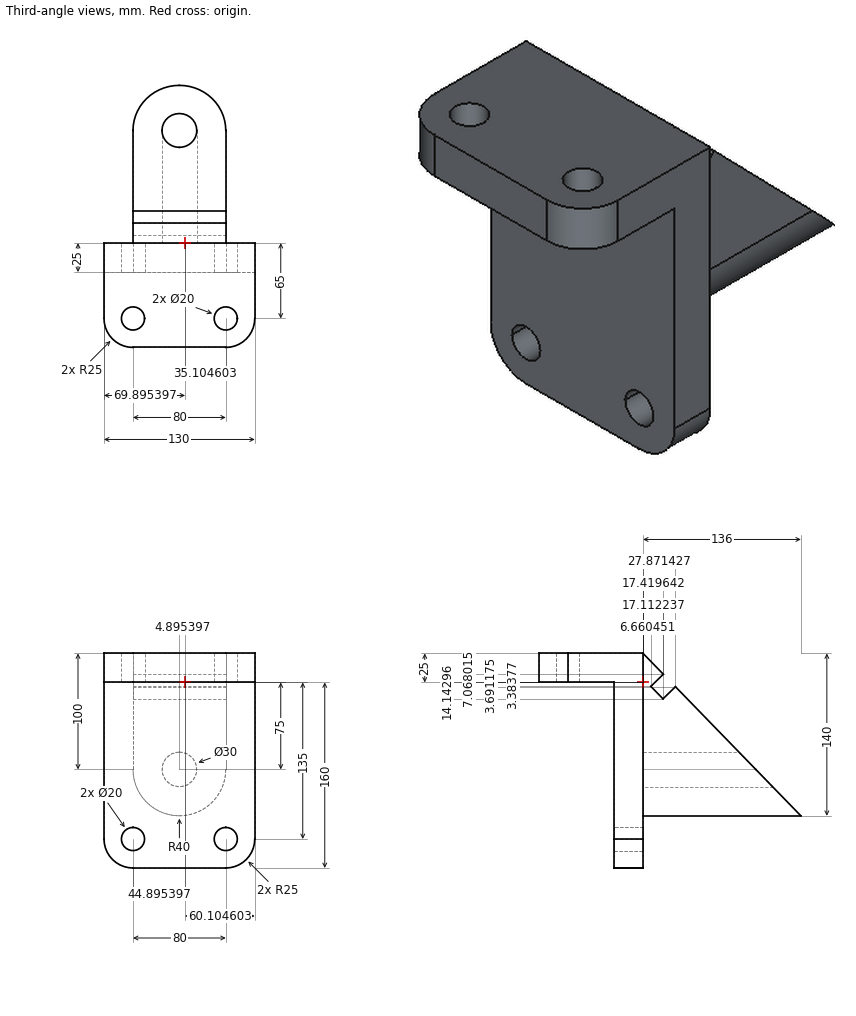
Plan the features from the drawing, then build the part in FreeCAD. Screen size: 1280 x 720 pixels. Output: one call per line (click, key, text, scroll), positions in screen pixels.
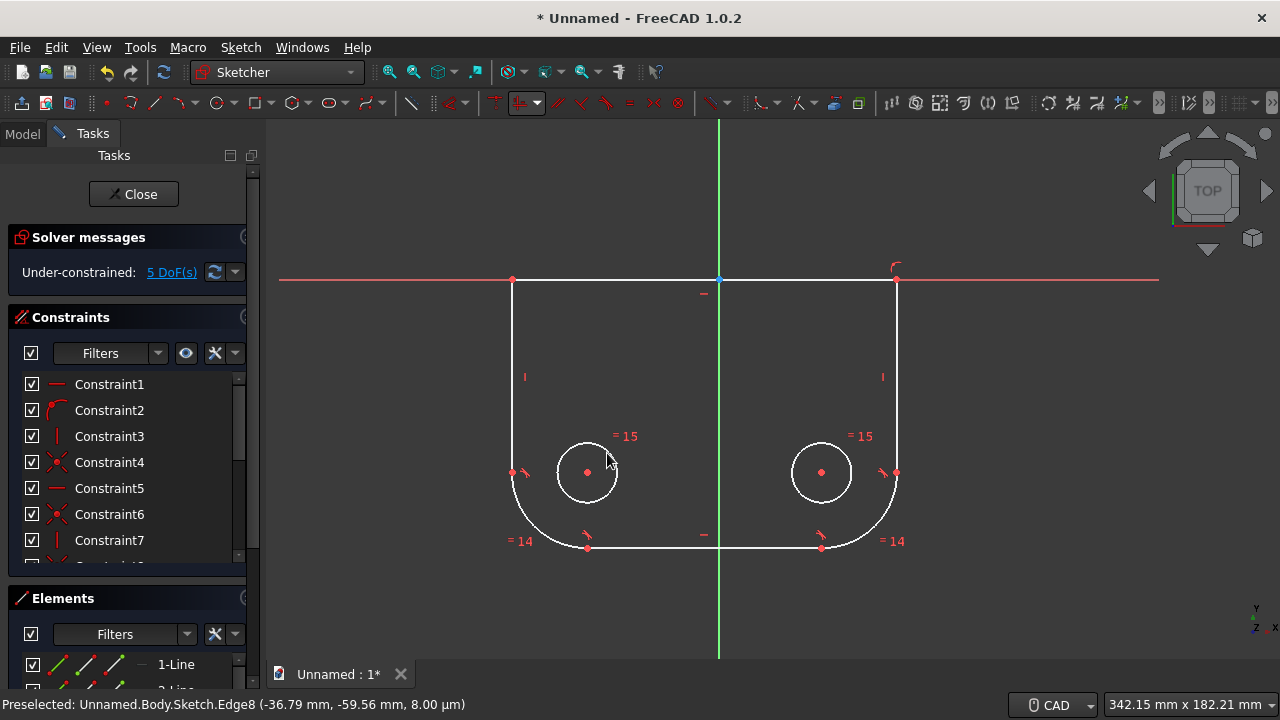
click(856, 540)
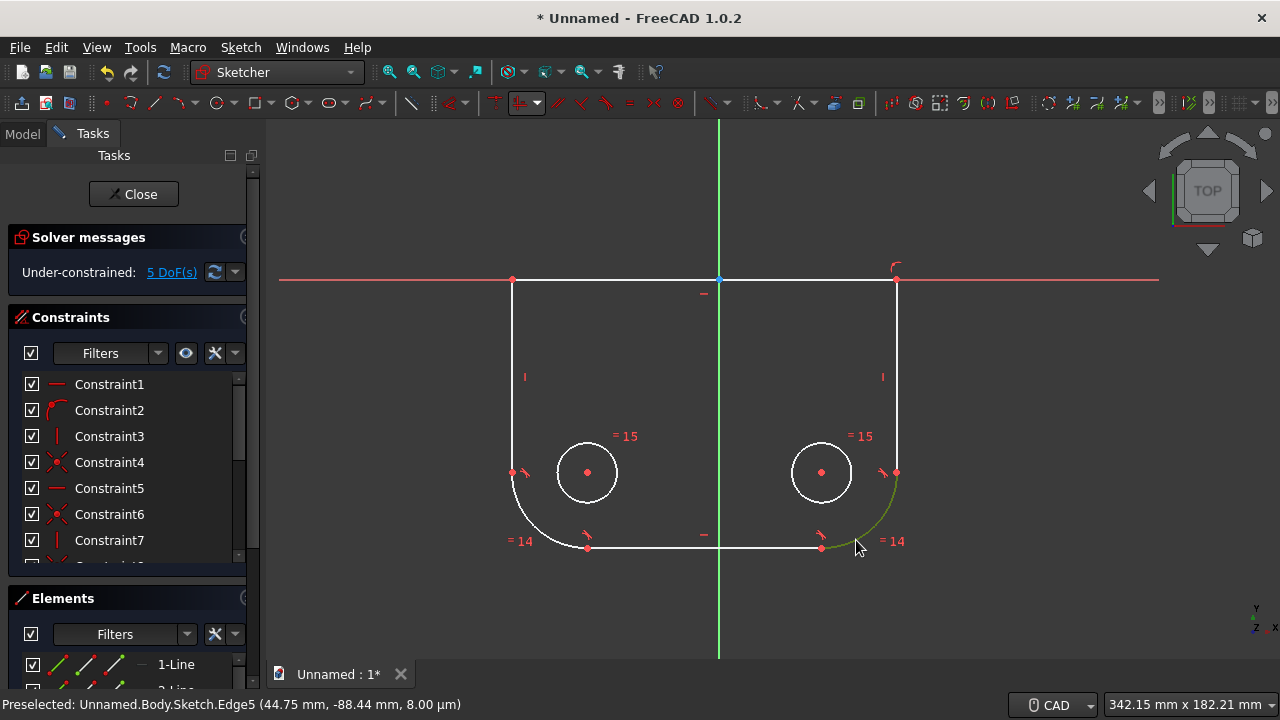
click(468, 104)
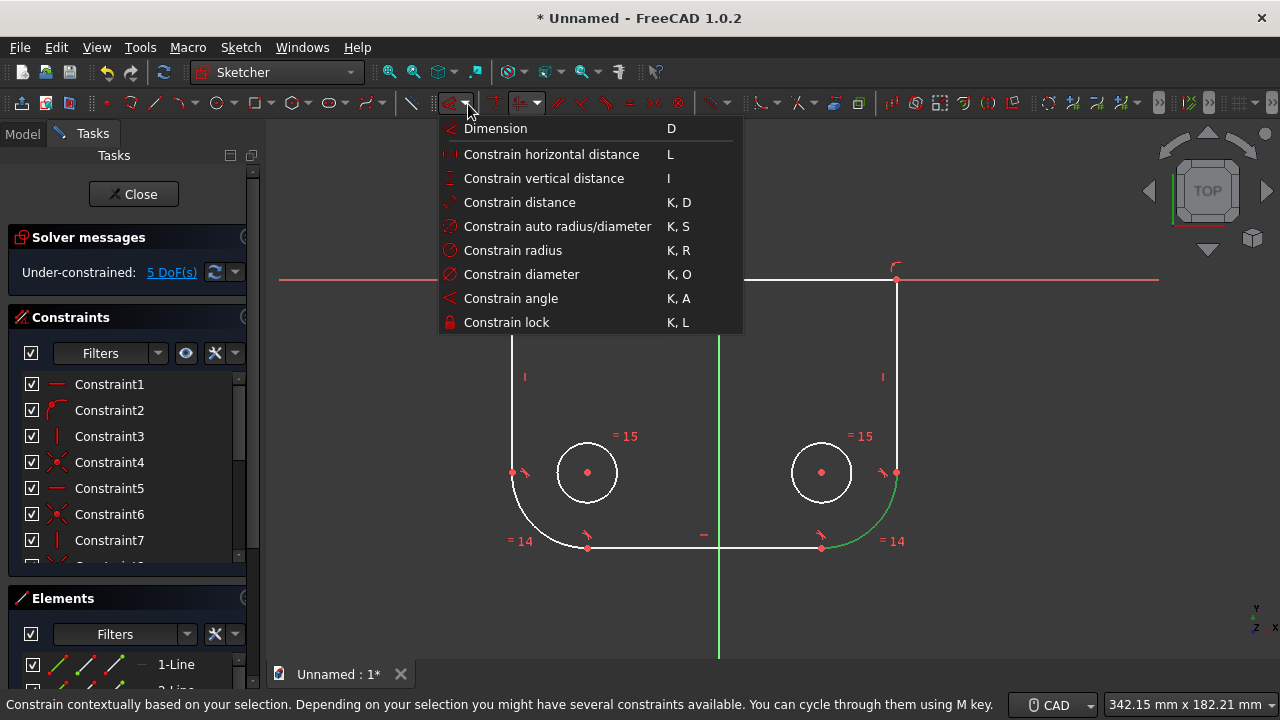
click(591, 250)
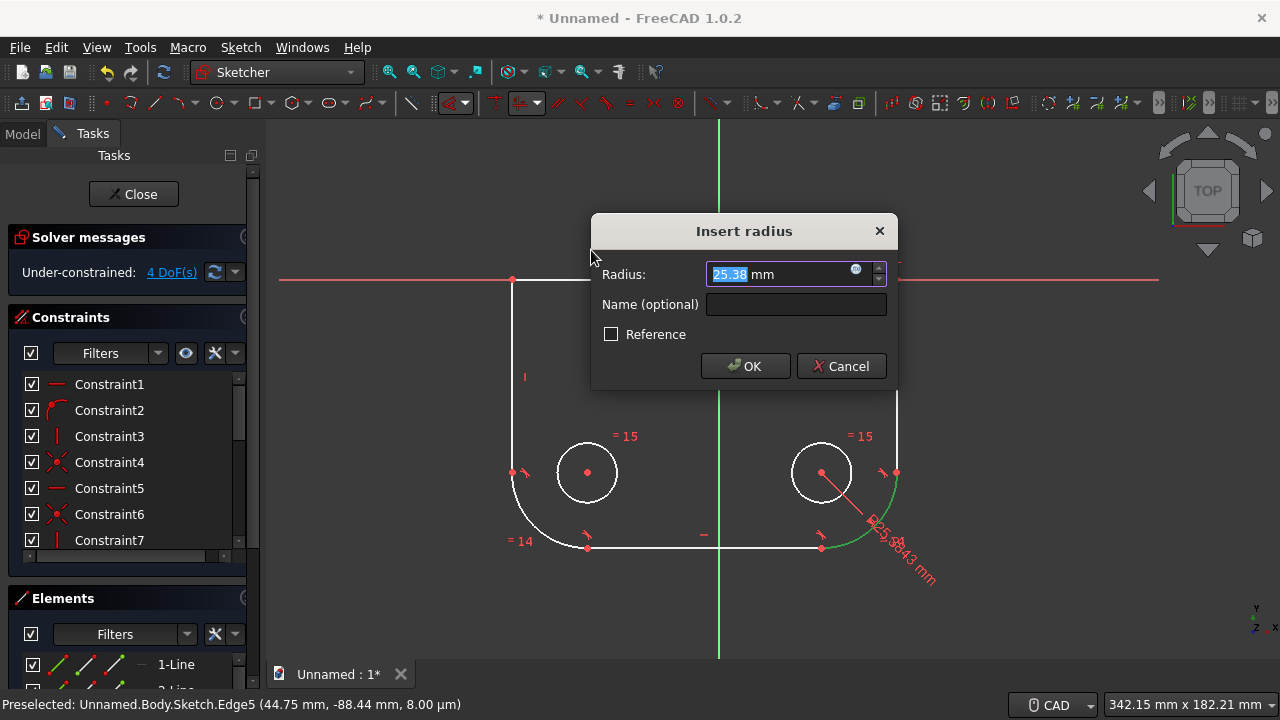
text(25)
key(Return)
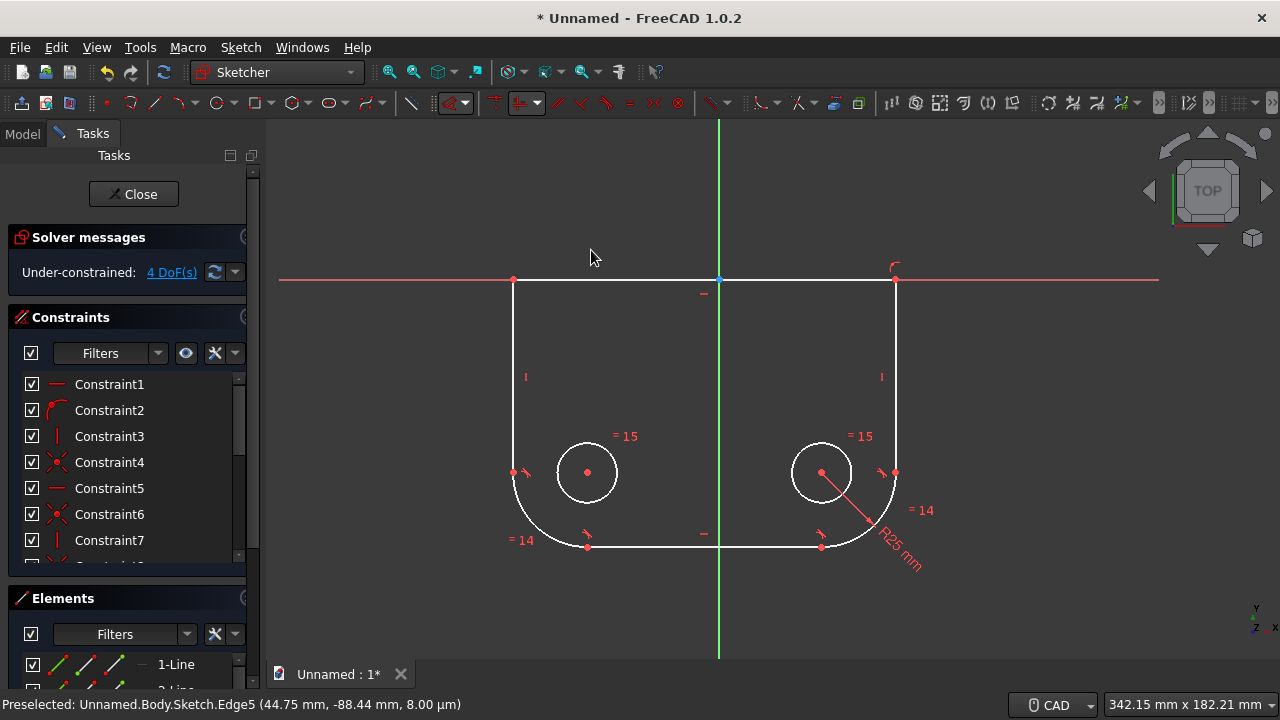
click(843, 452)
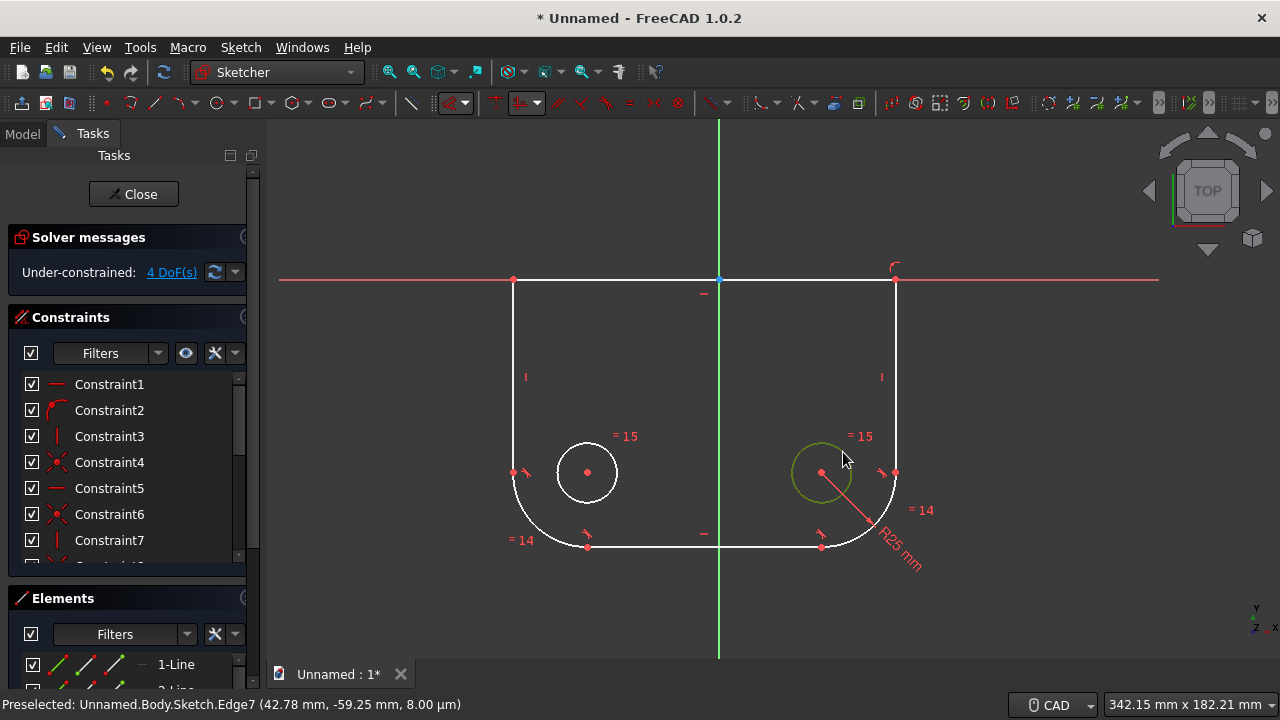
key(k)
key(o)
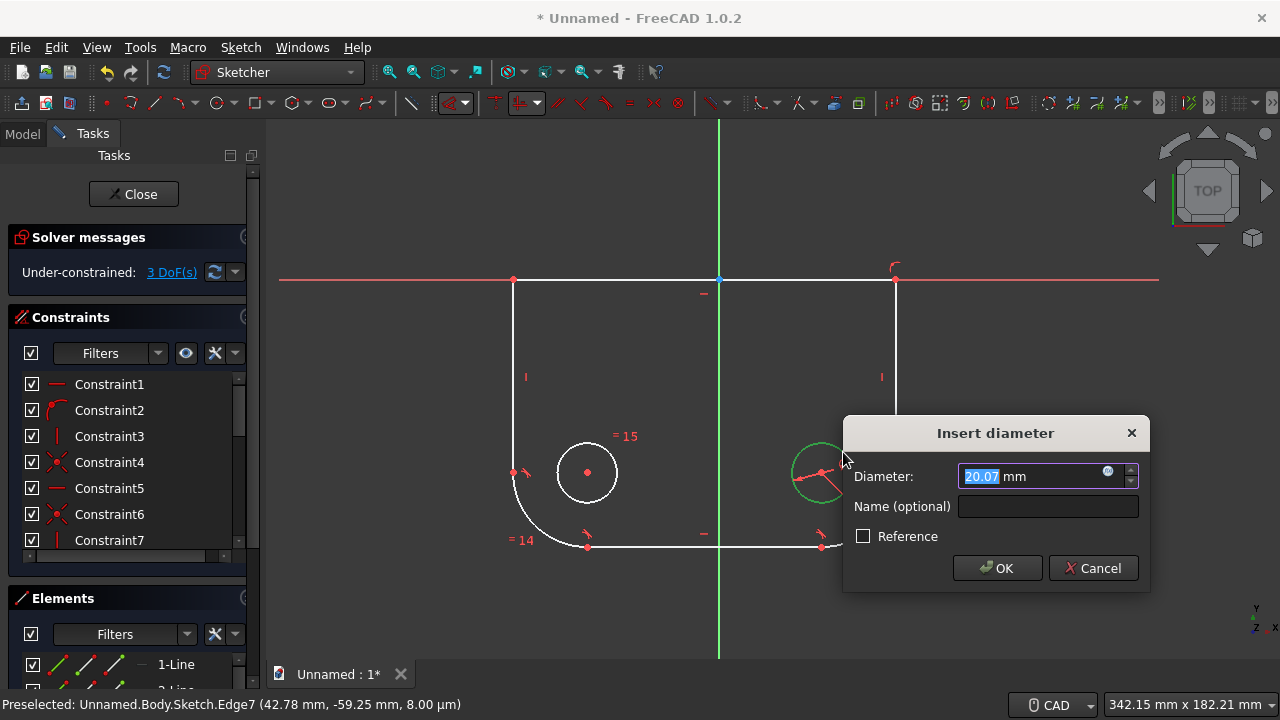
text(20)
key(Return)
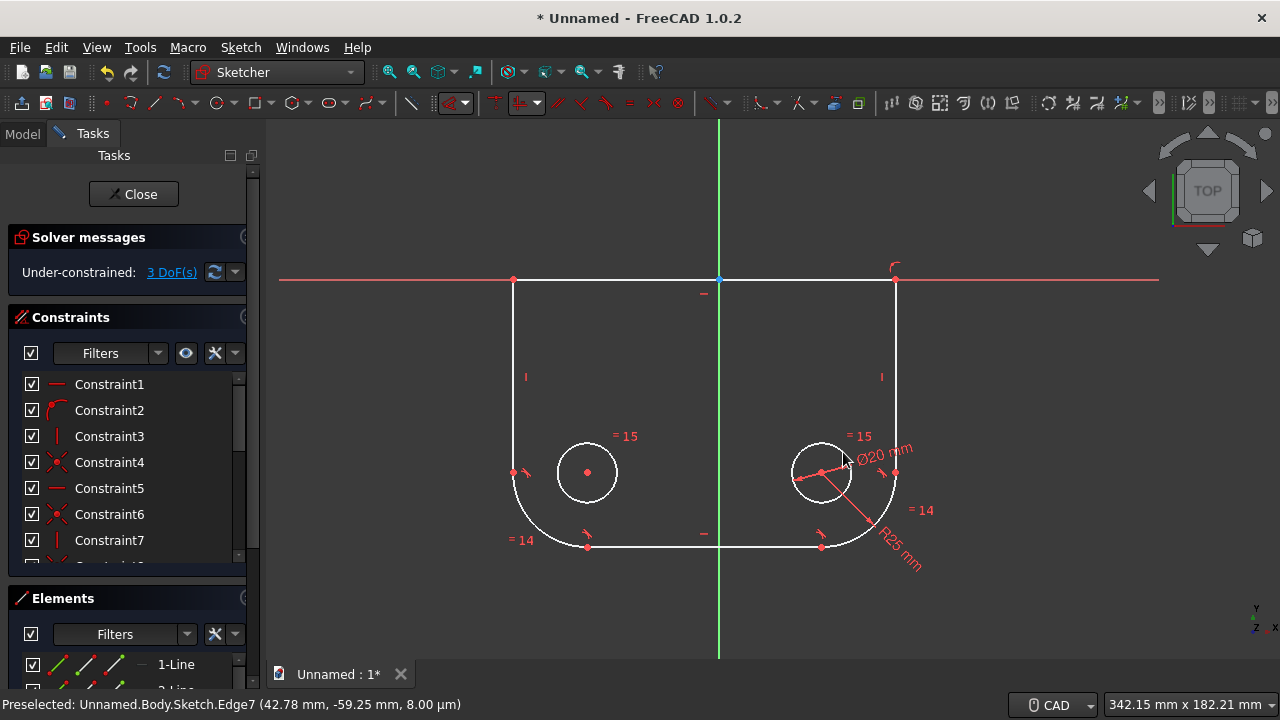
click(658, 547)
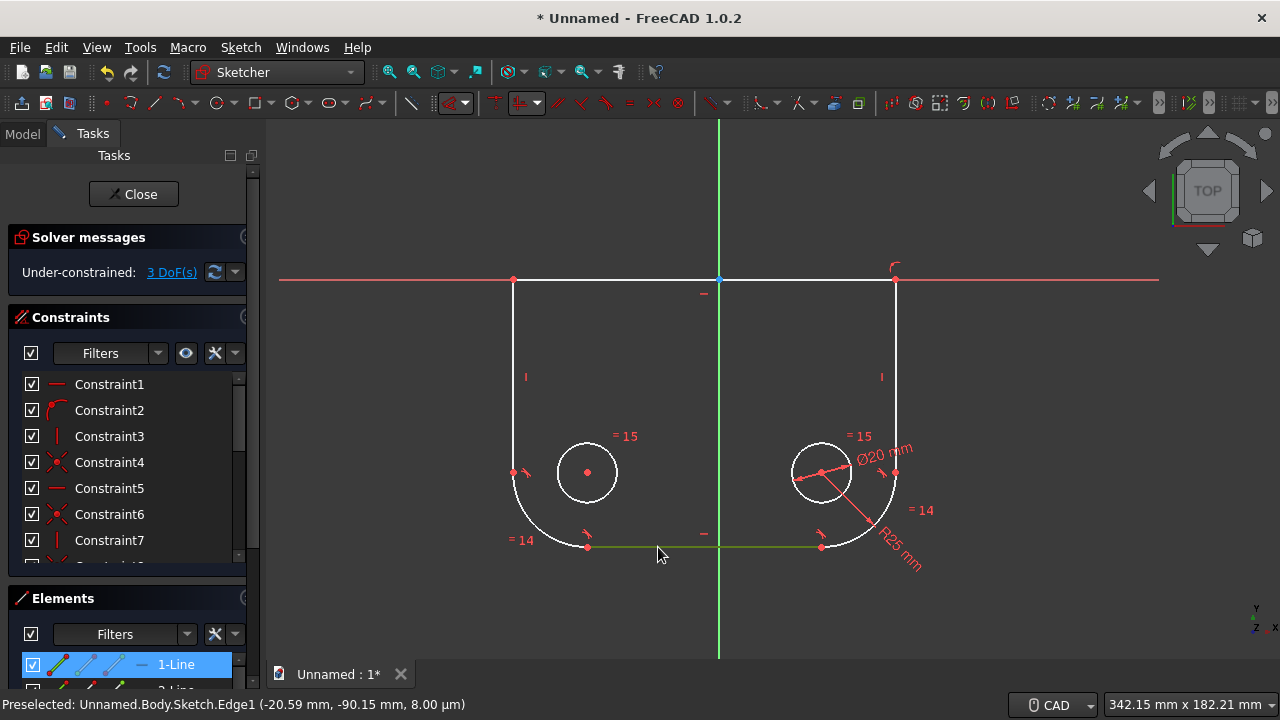
click(468, 104)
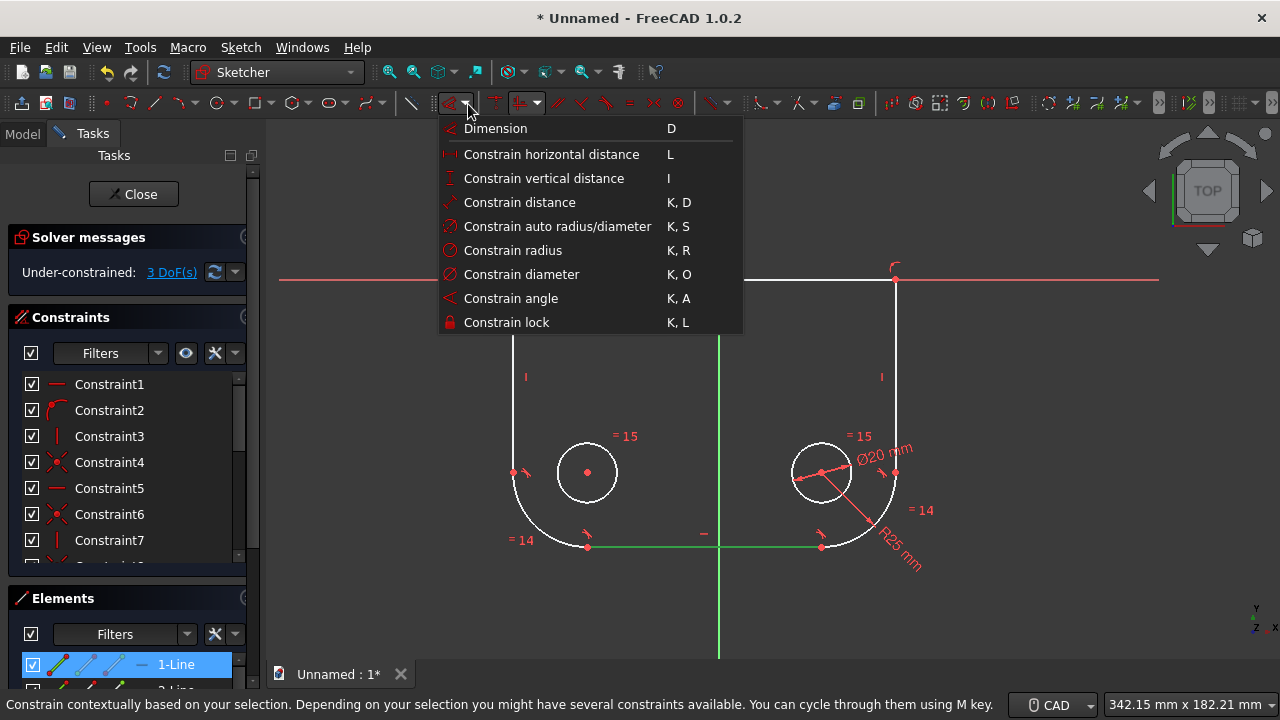
click(591, 154)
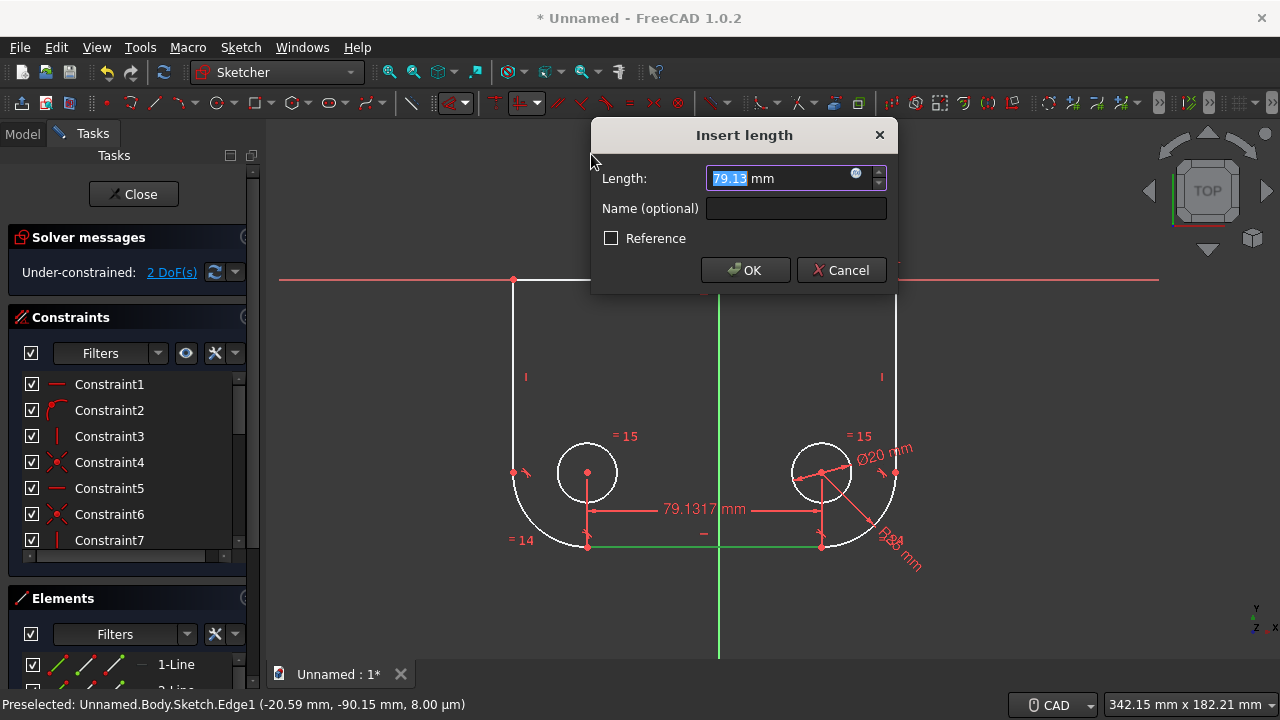
text(80)
key(Return)